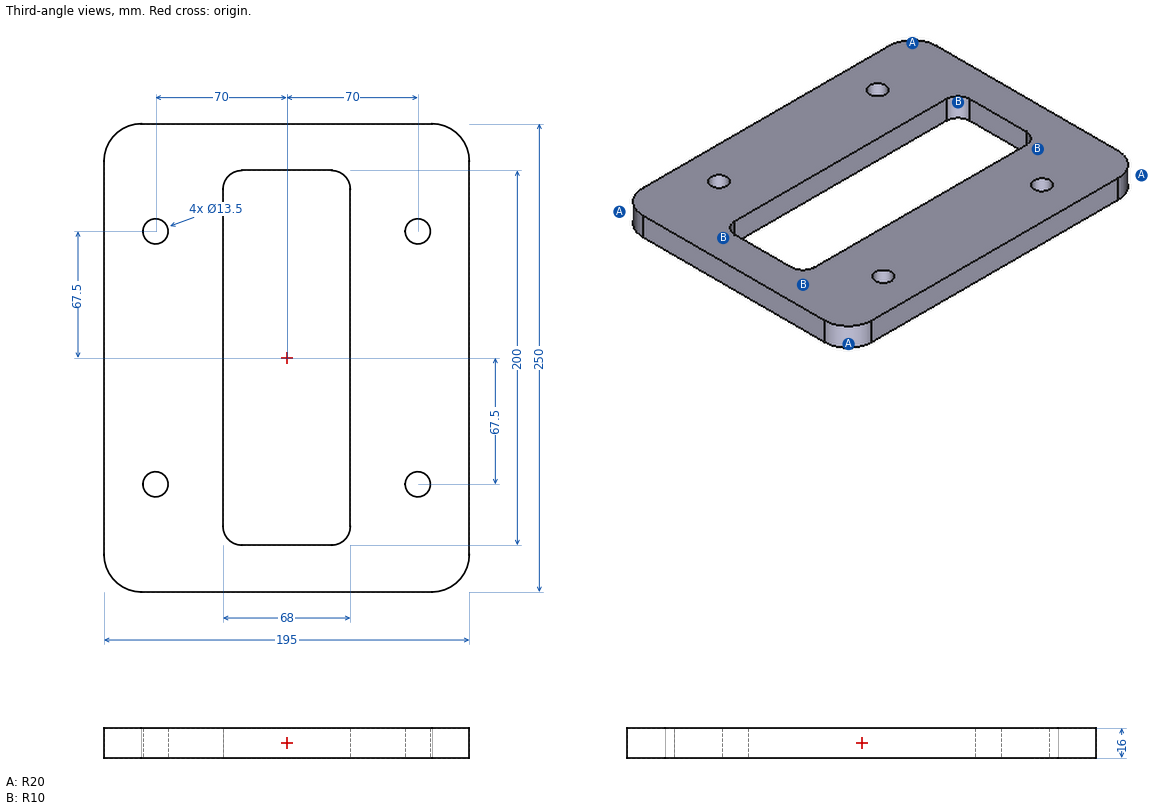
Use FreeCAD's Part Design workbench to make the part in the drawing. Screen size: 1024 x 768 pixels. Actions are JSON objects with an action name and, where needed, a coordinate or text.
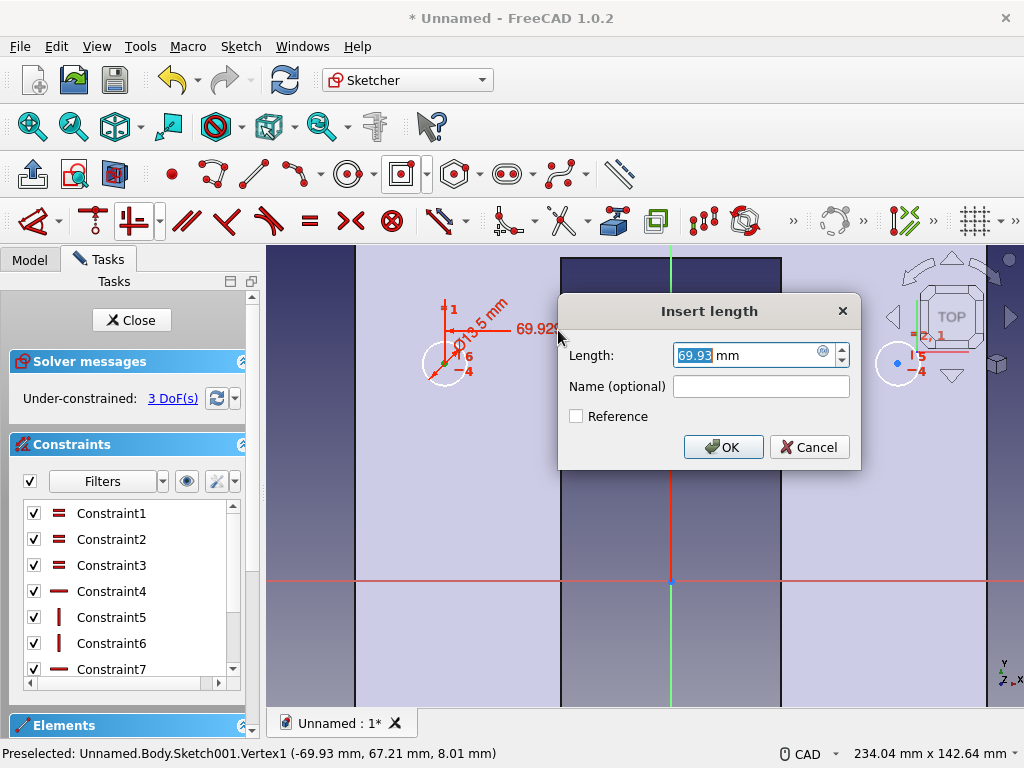
{"action": "type", "text": "70"}
{"action": "key", "text": "Return"}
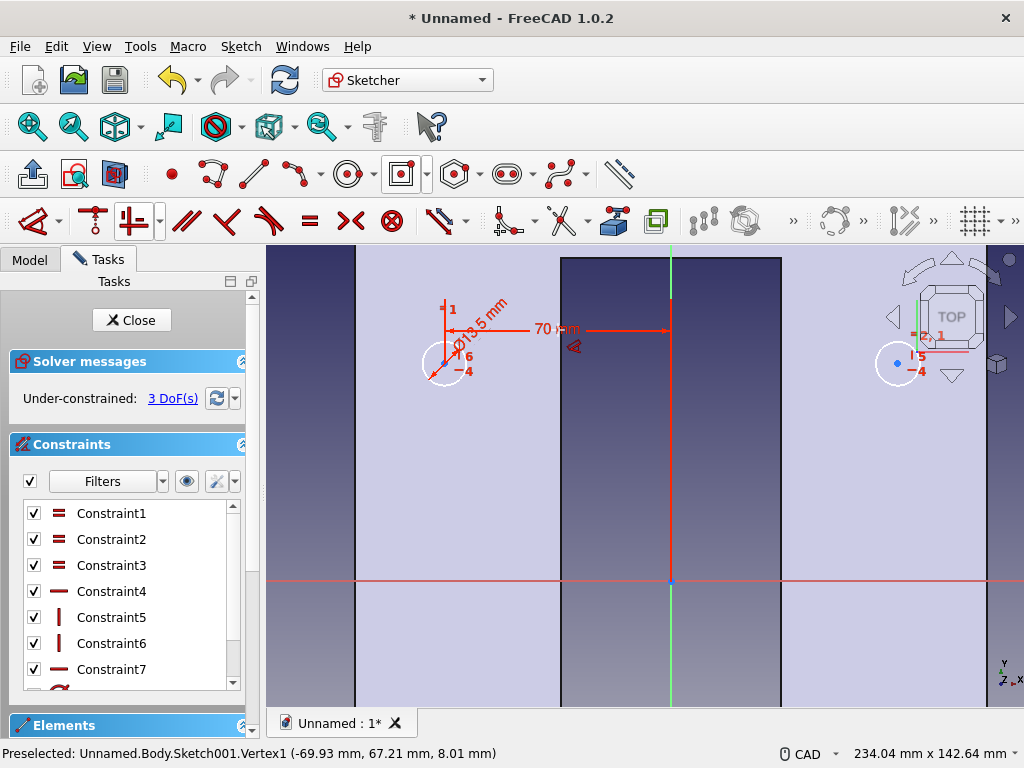
{"action": "scroll", "coordinate": [461, 348], "scroll_direction": "down", "scroll_amount": 3}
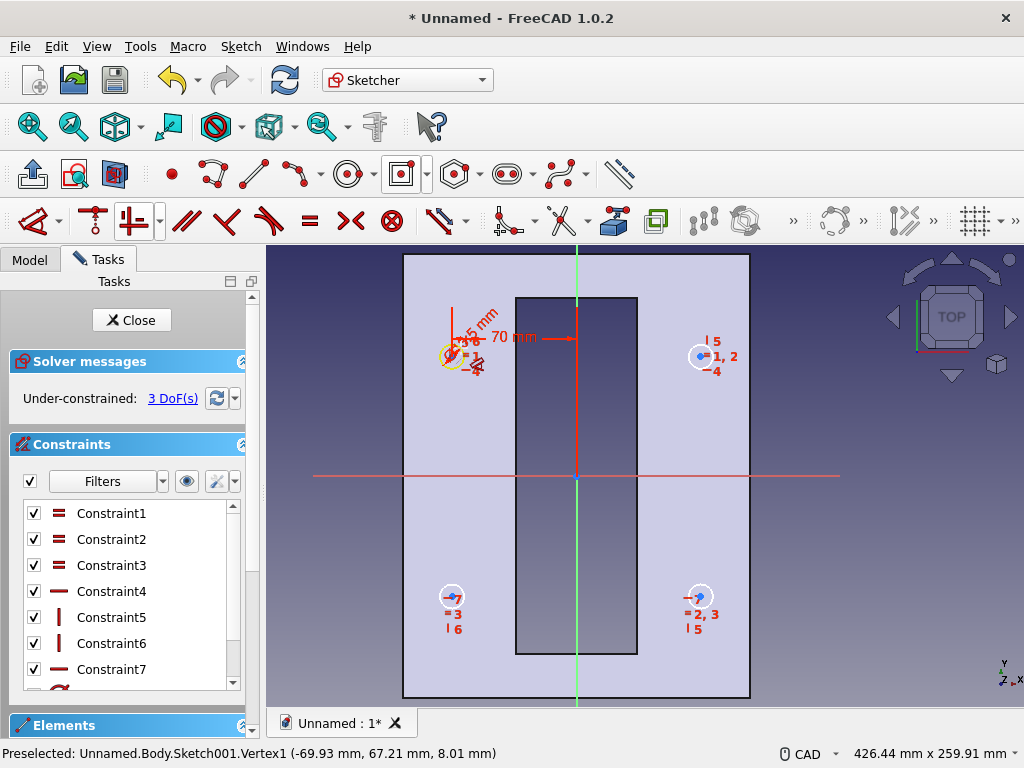
{"action": "left_click", "coordinate": [701, 357]}
{"action": "left_click", "coordinate": [639, 323]}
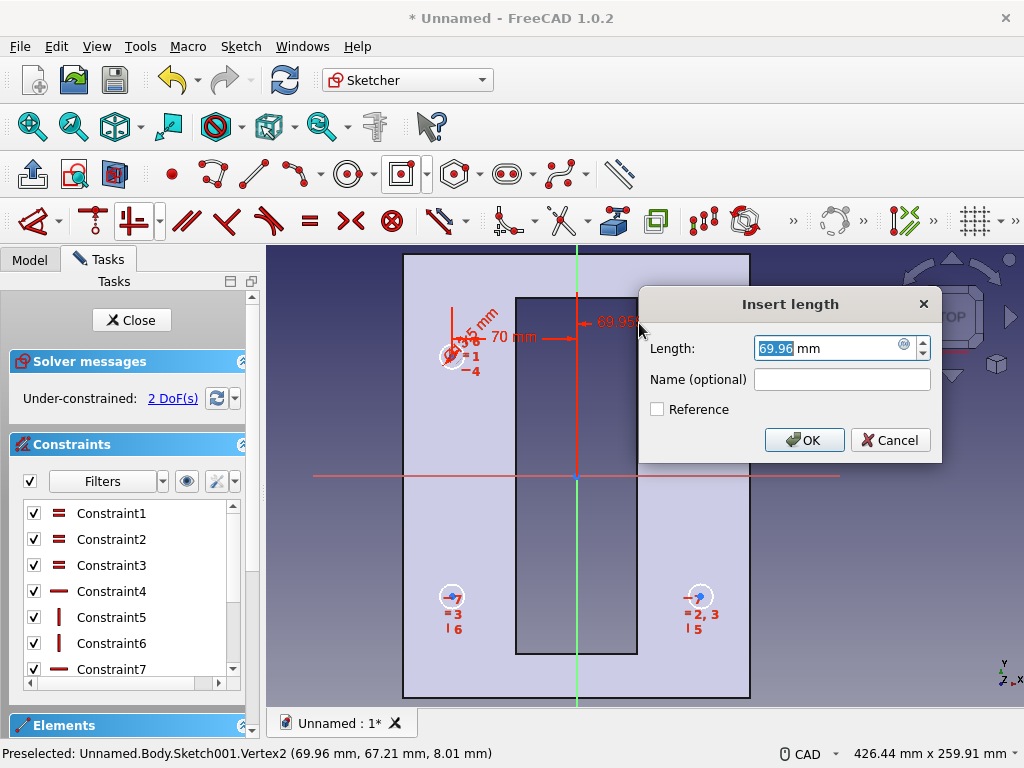
{"action": "type", "text": "70"}
{"action": "key", "text": "Return"}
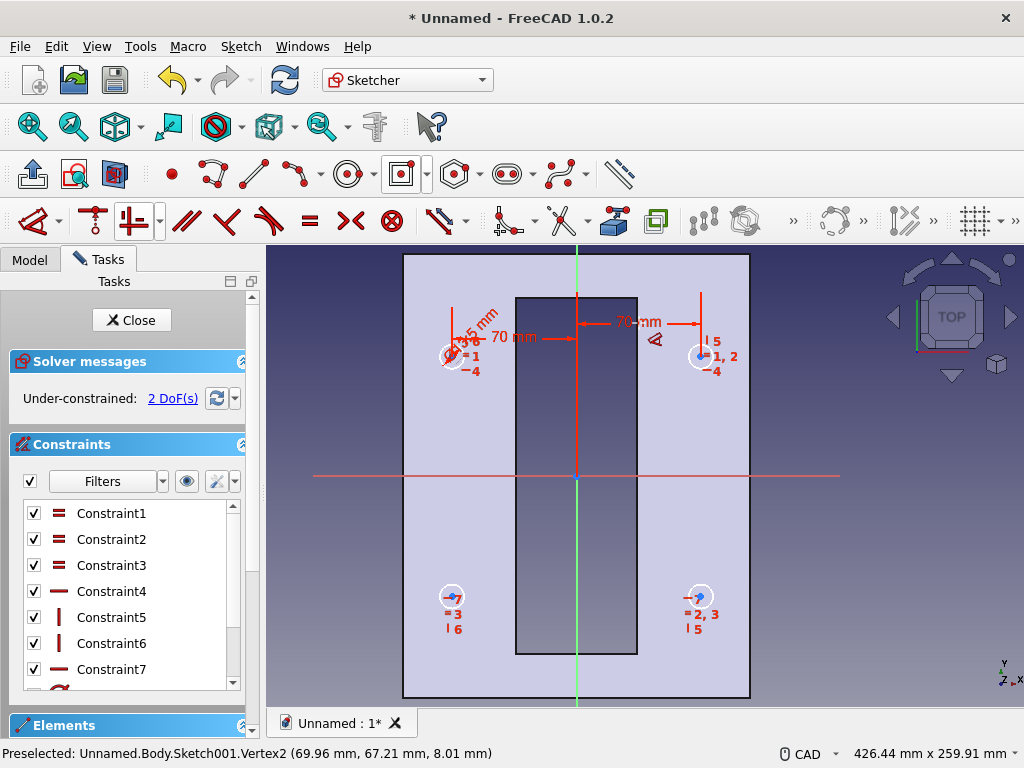
{"action": "left_click", "coordinate": [452, 357]}
{"action": "left_click", "coordinate": [418, 416]}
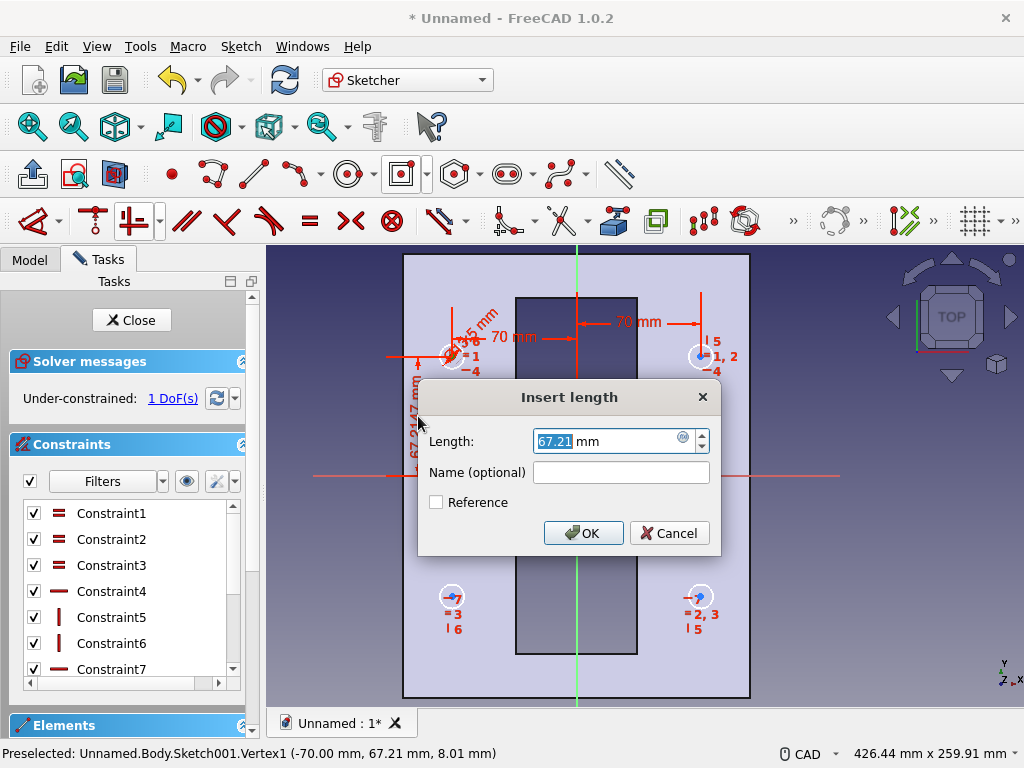
{"action": "type", "text": "67.5"}
{"action": "key", "text": "Return"}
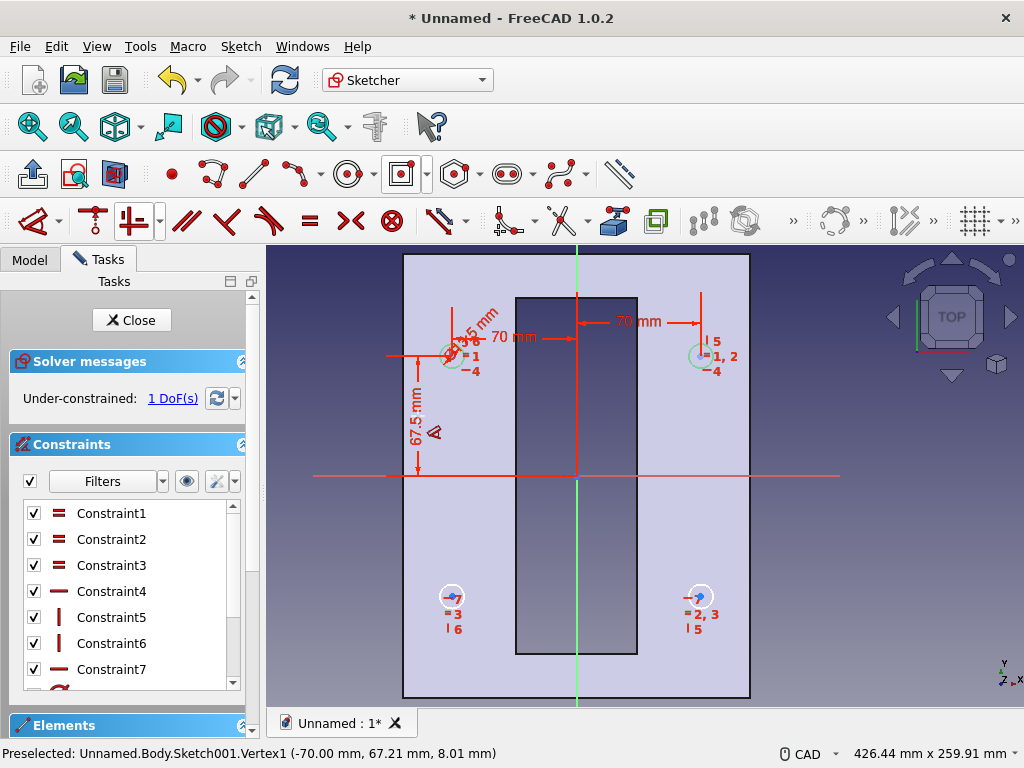
{"action": "left_click", "coordinate": [701, 597]}
{"action": "left_click", "coordinate": [735, 536]}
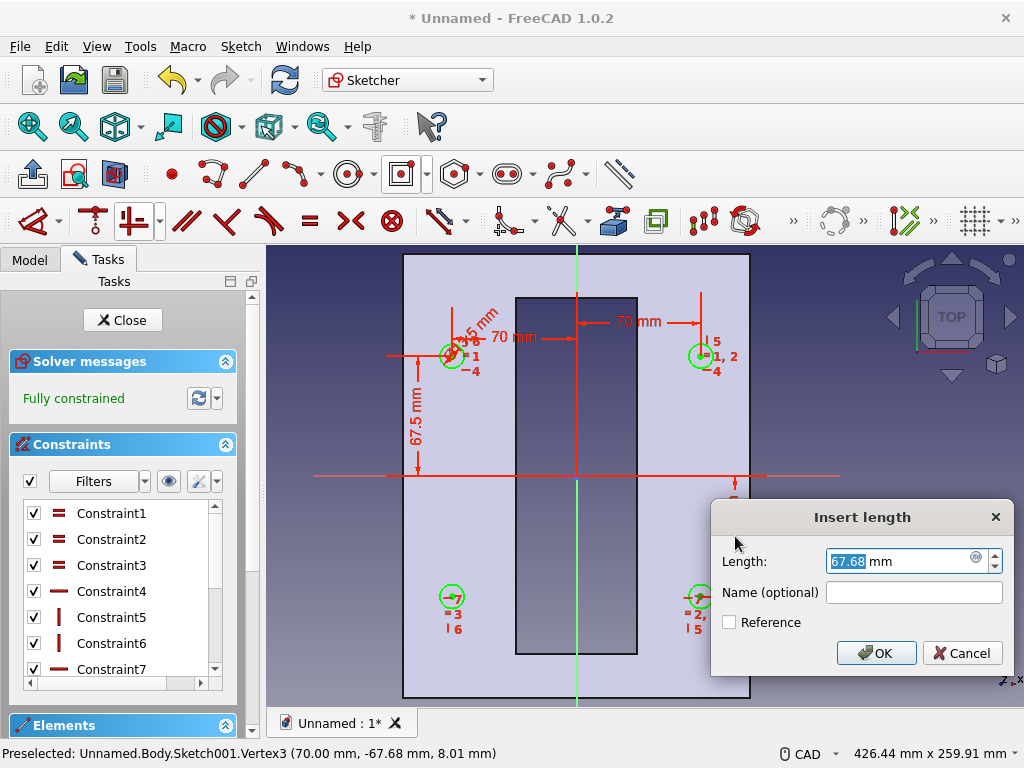
{"action": "type", "text": "67.5"}
{"action": "key", "text": "Return"}
{"action": "key", "text": "Escape"}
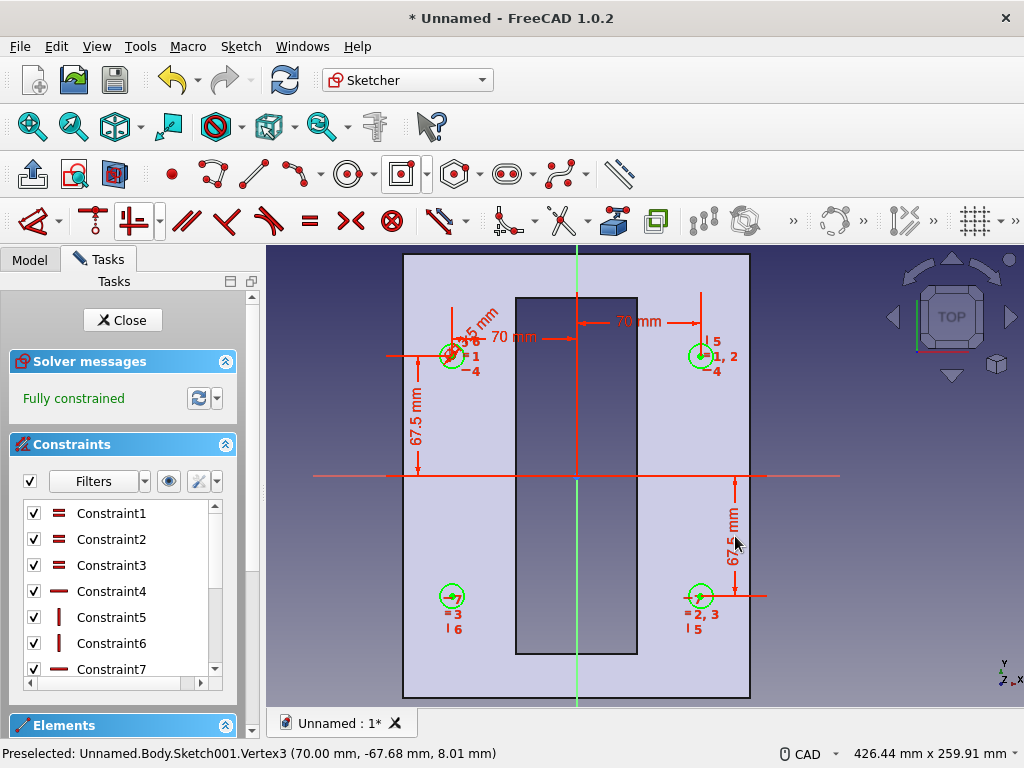
{"action": "left_click", "coordinate": [123, 320]}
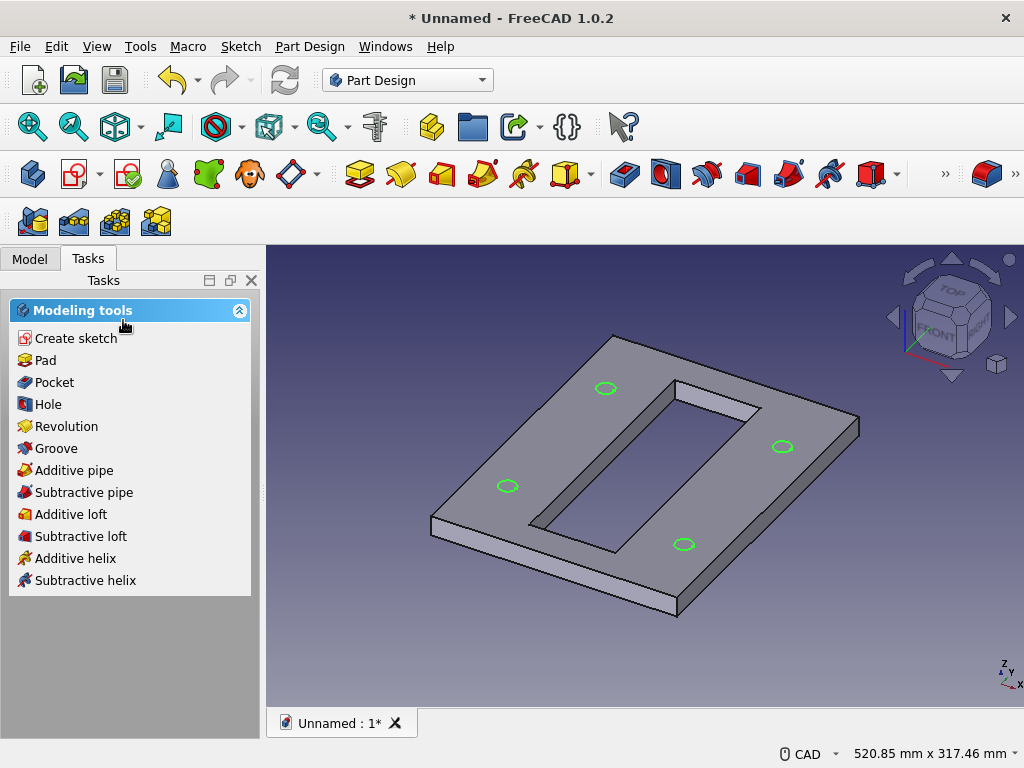
{"action": "left_click", "coordinate": [625, 174]}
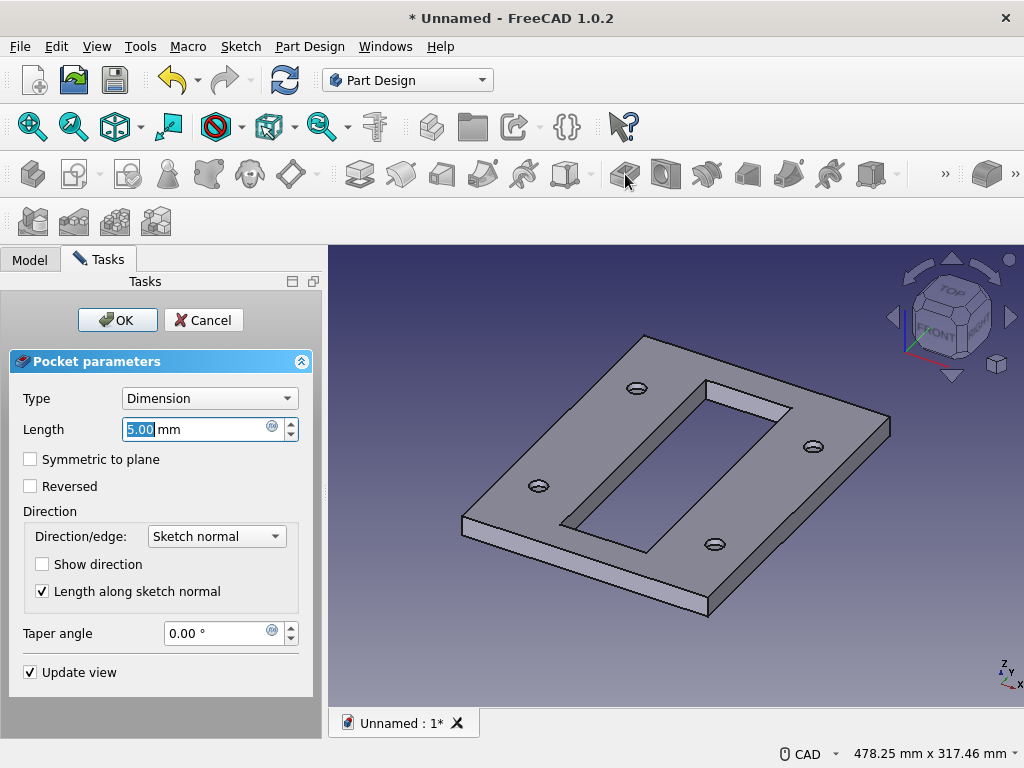
{"action": "left_click", "coordinate": [210, 398]}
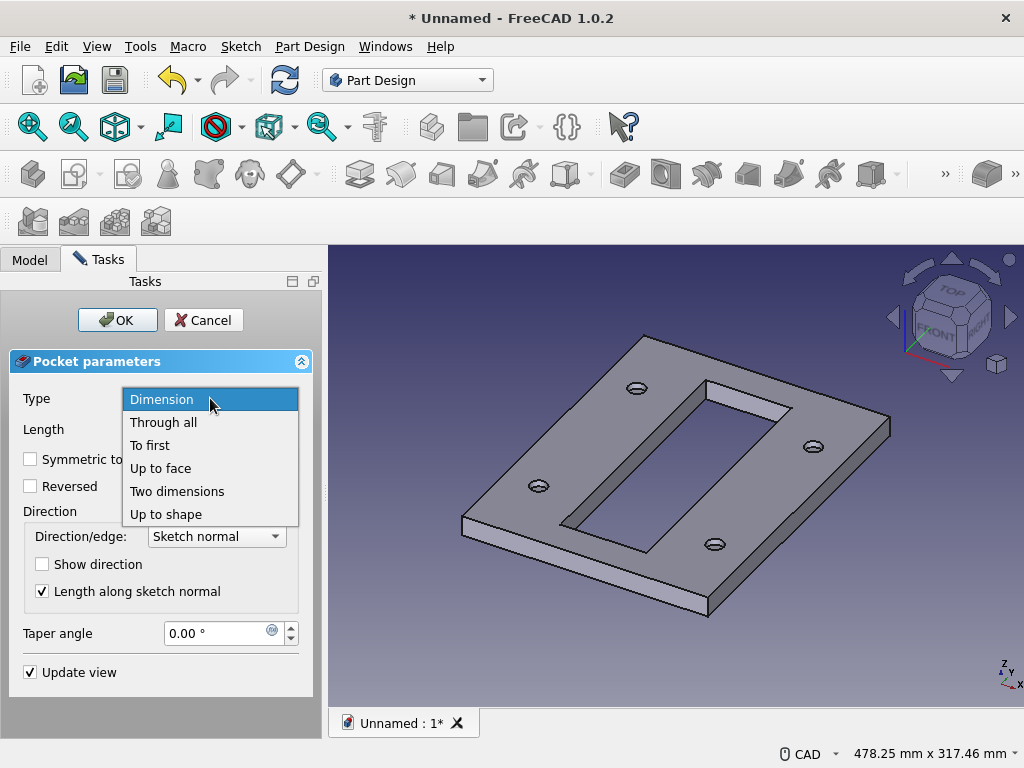
{"action": "left_click", "coordinate": [208, 422]}